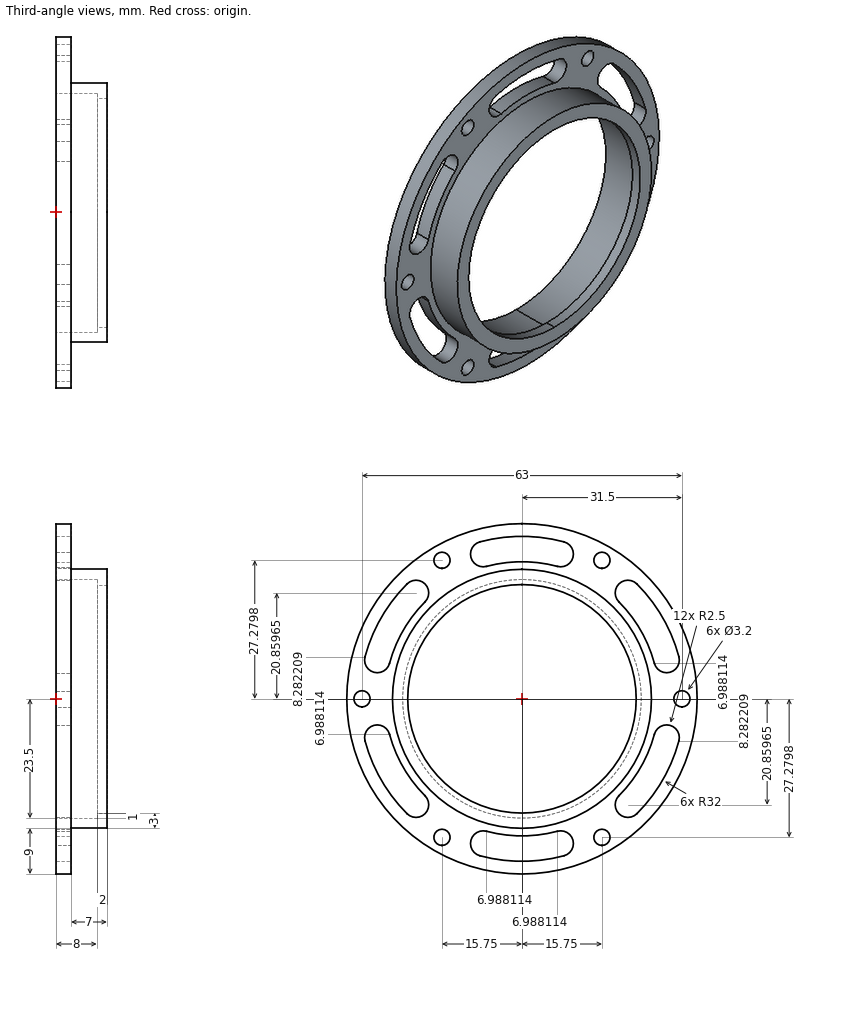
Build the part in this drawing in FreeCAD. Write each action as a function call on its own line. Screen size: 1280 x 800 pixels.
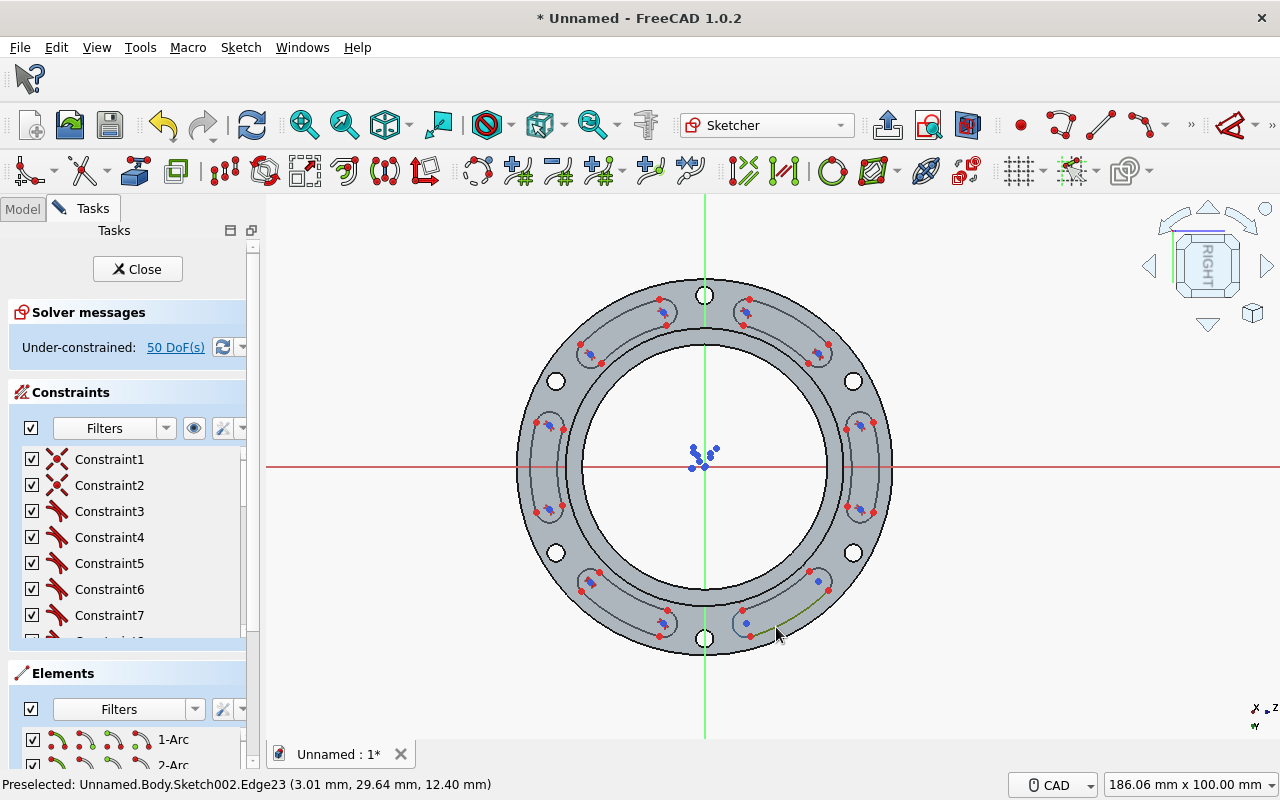
key(t)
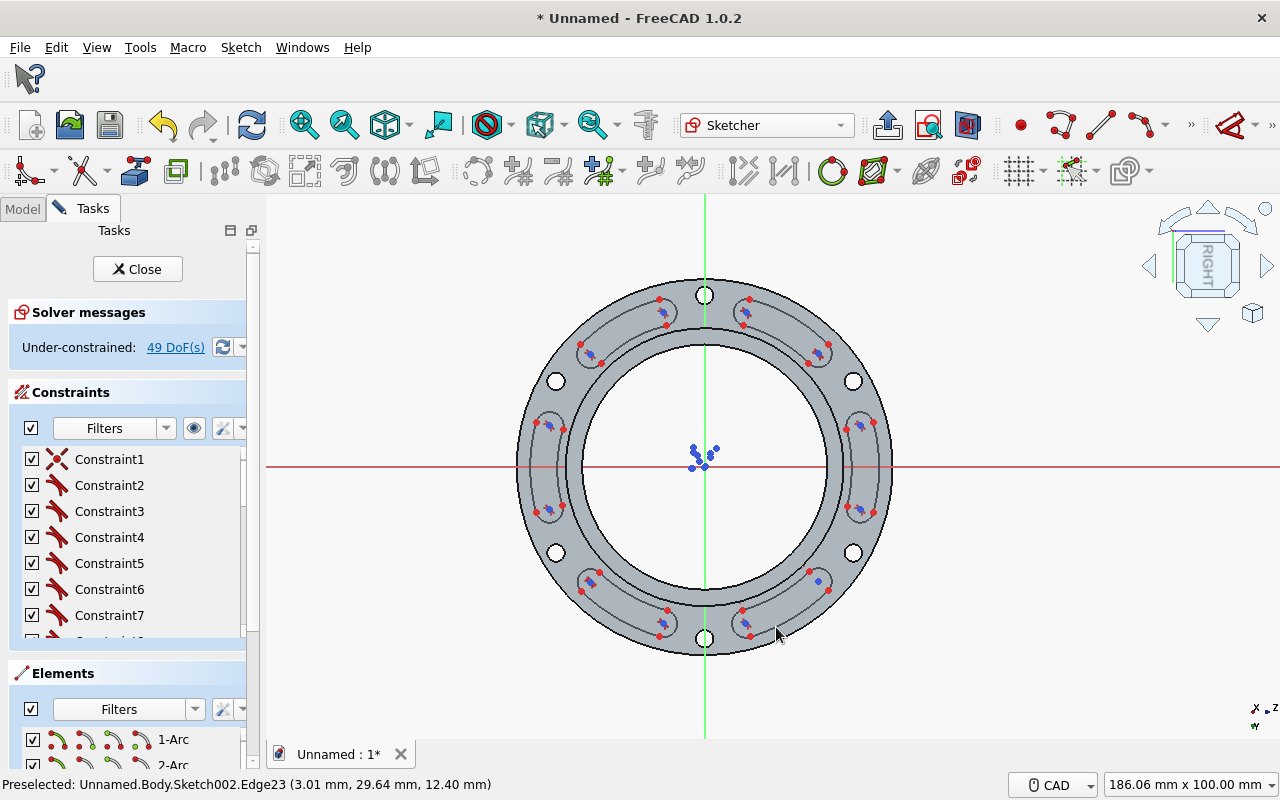
click(776, 627)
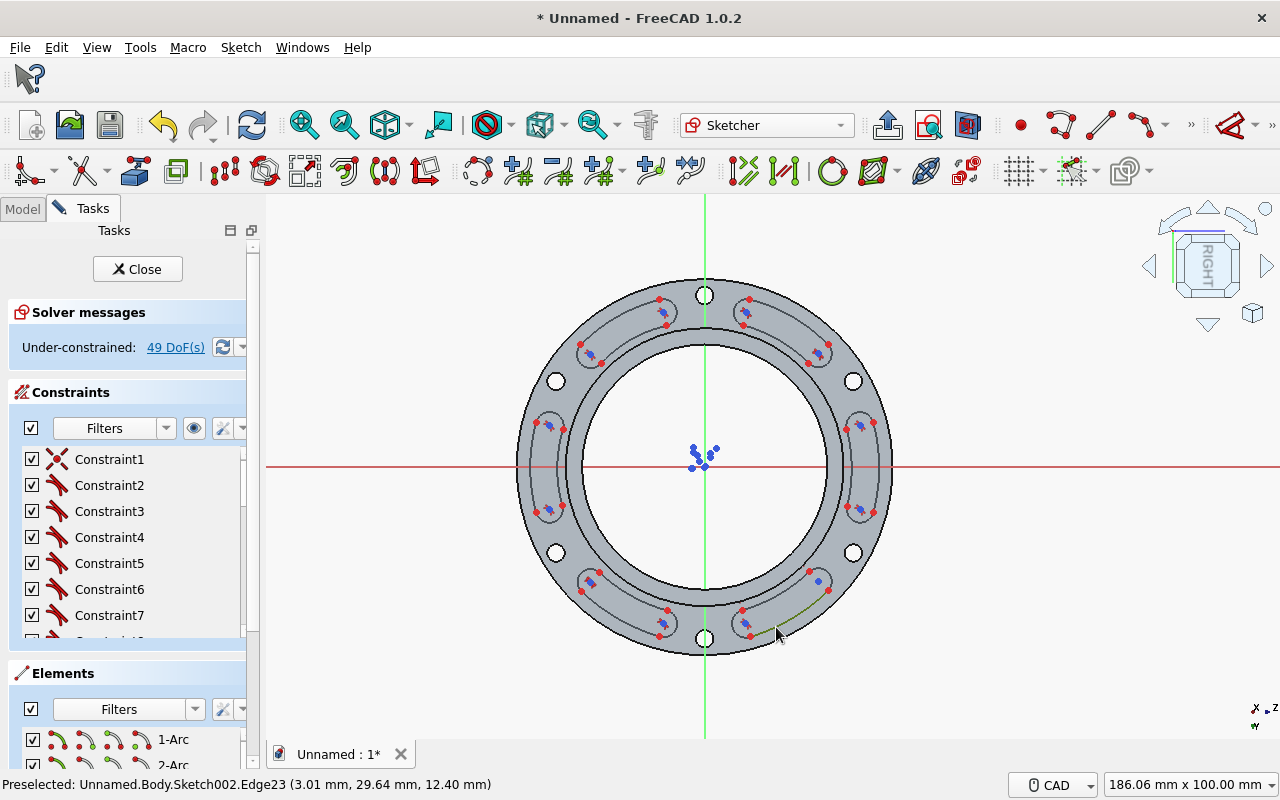
click(832, 579)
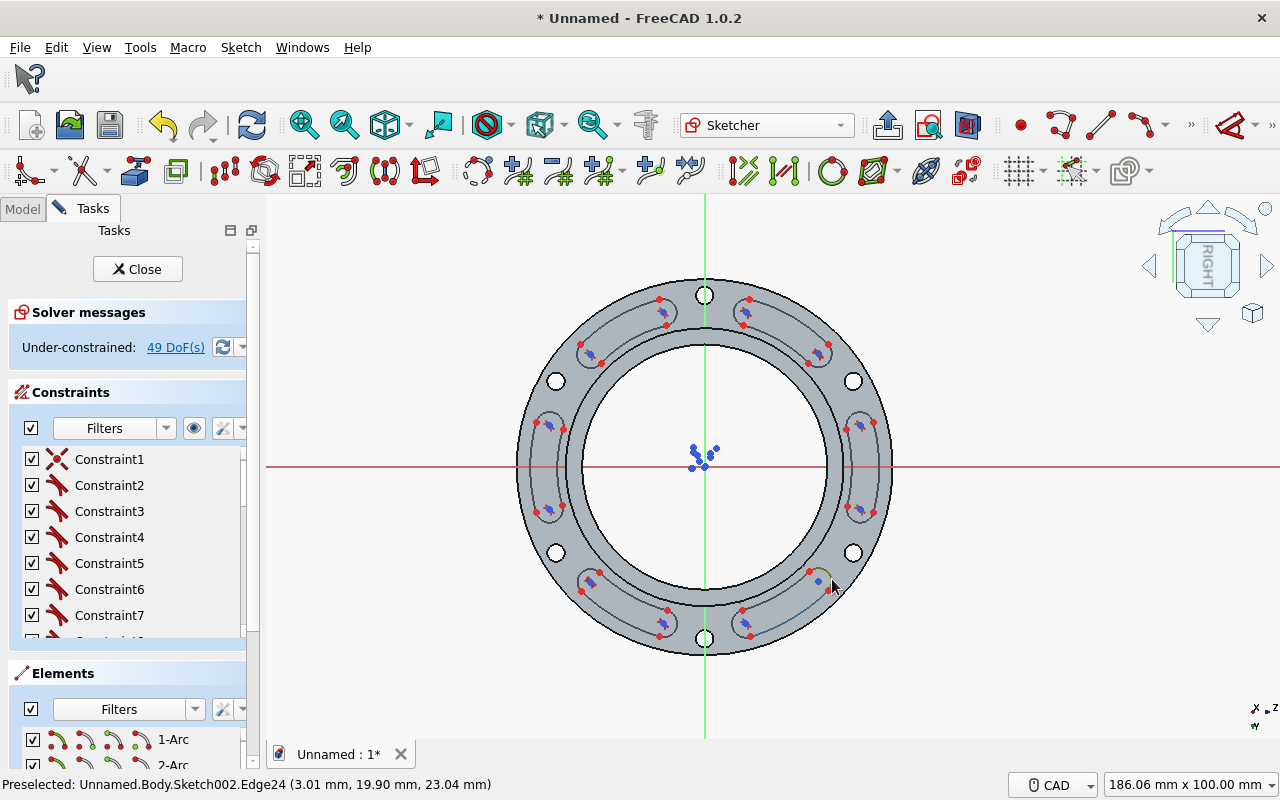
key(t)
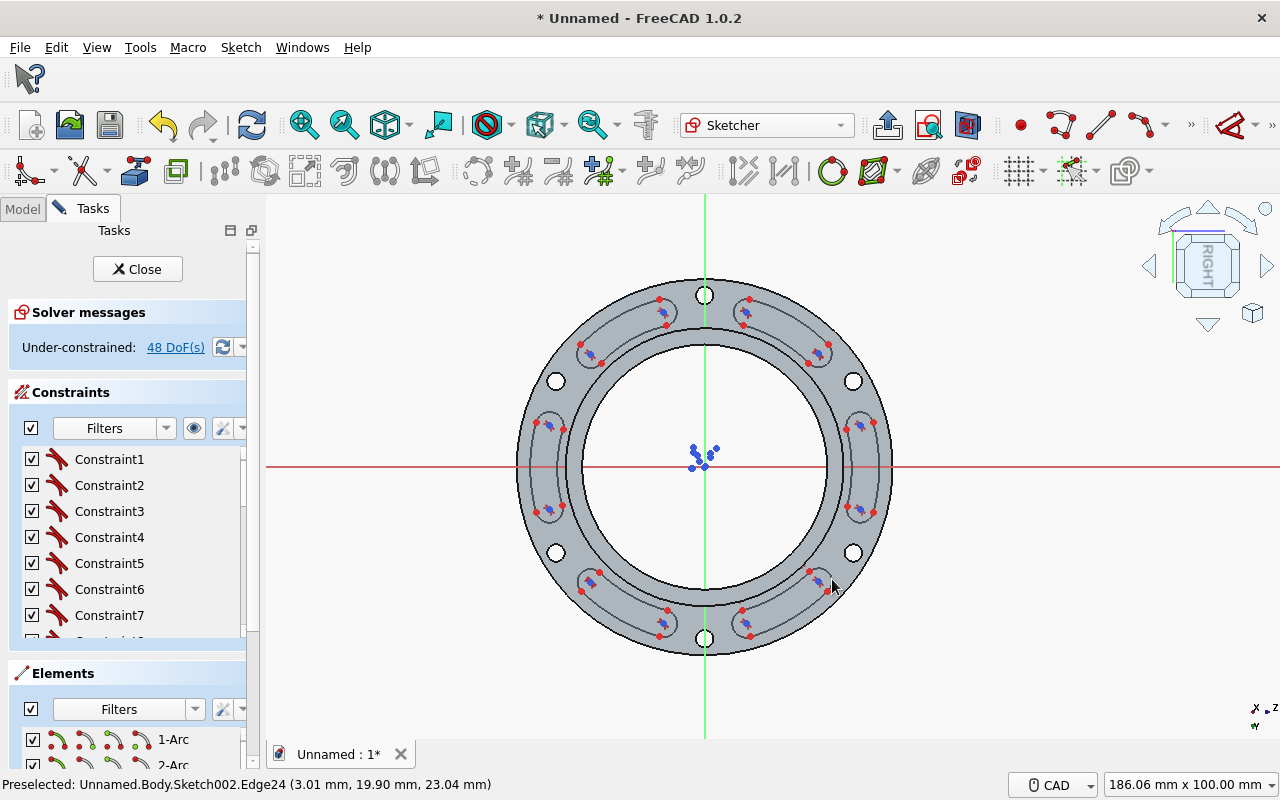
click(603, 609)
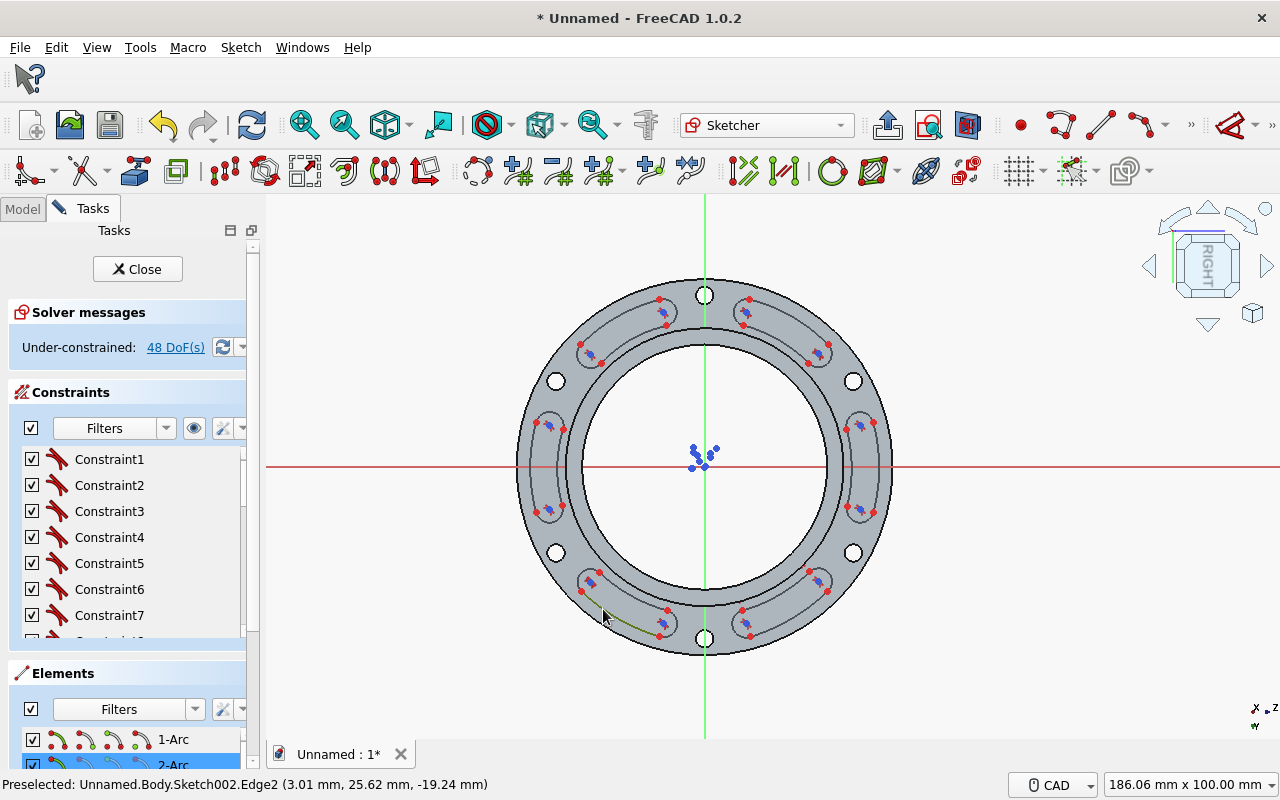
click(618, 587)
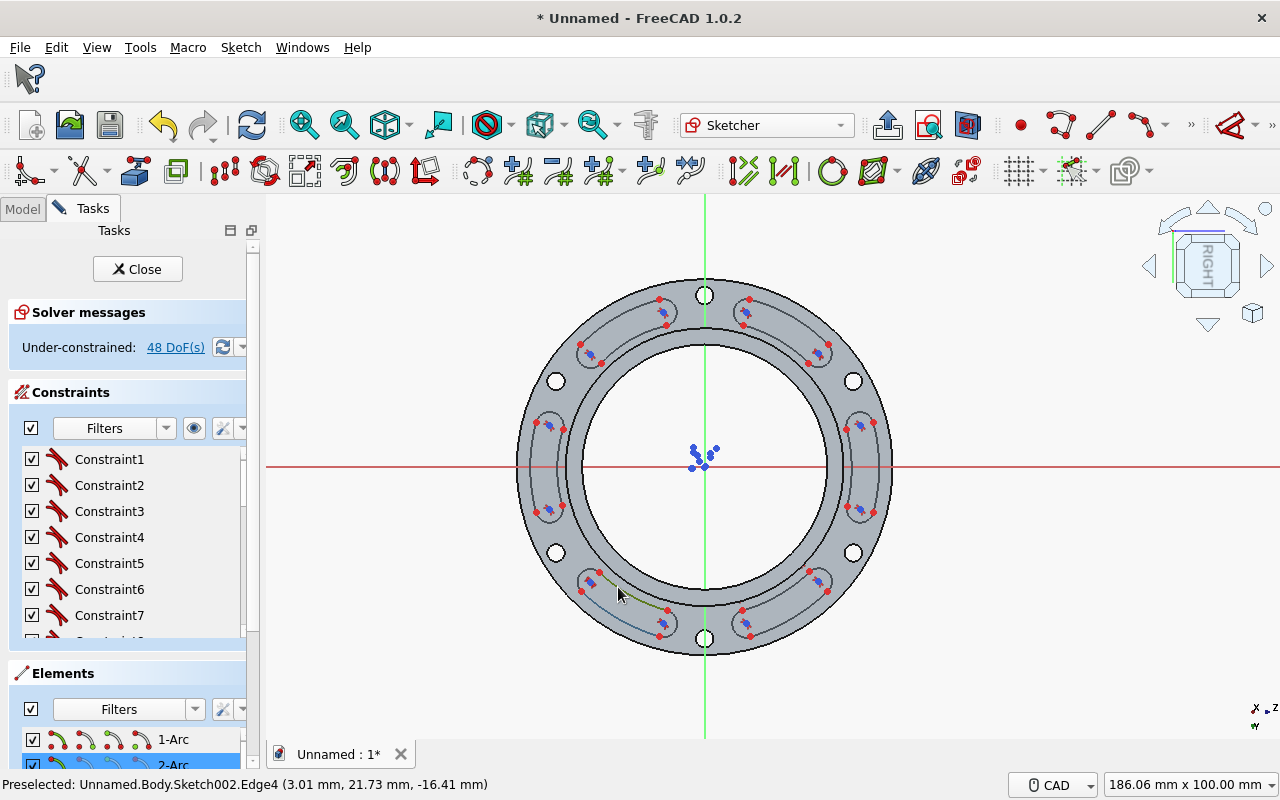
key(c)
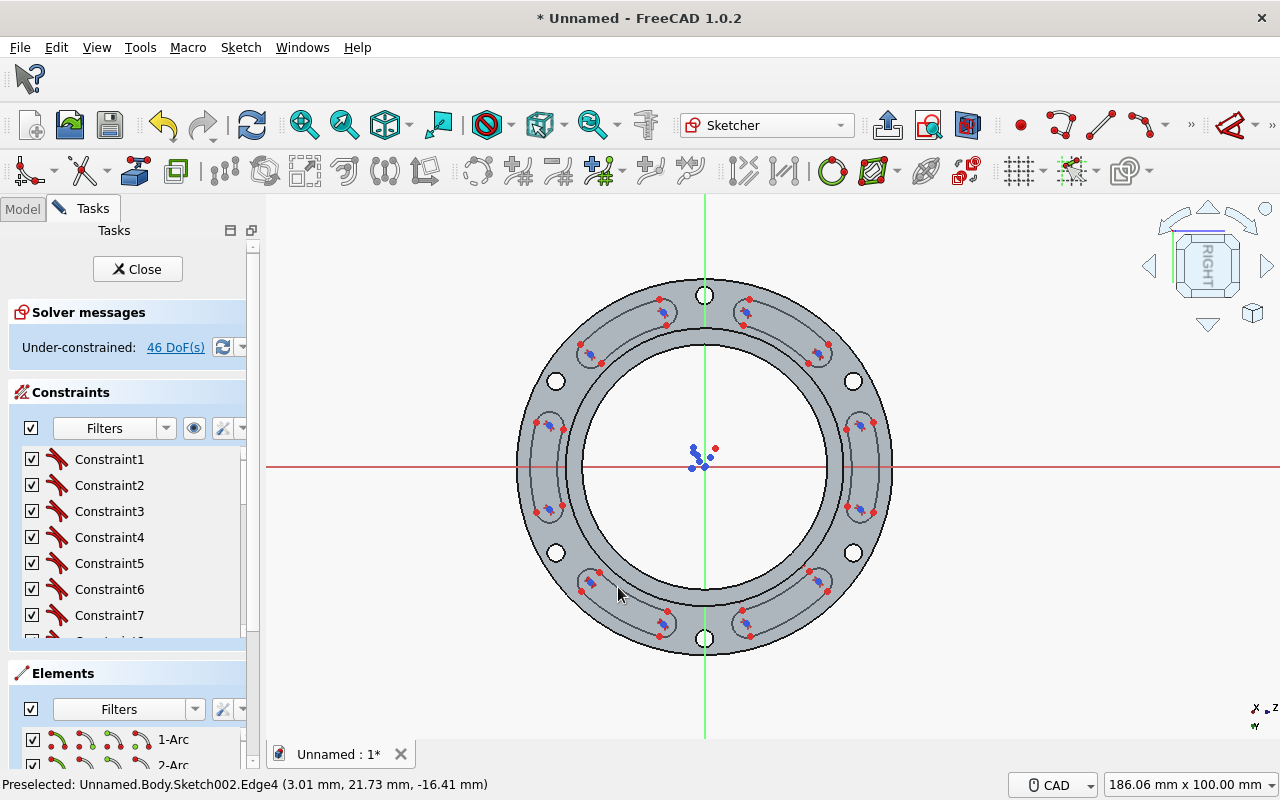
click(603, 609)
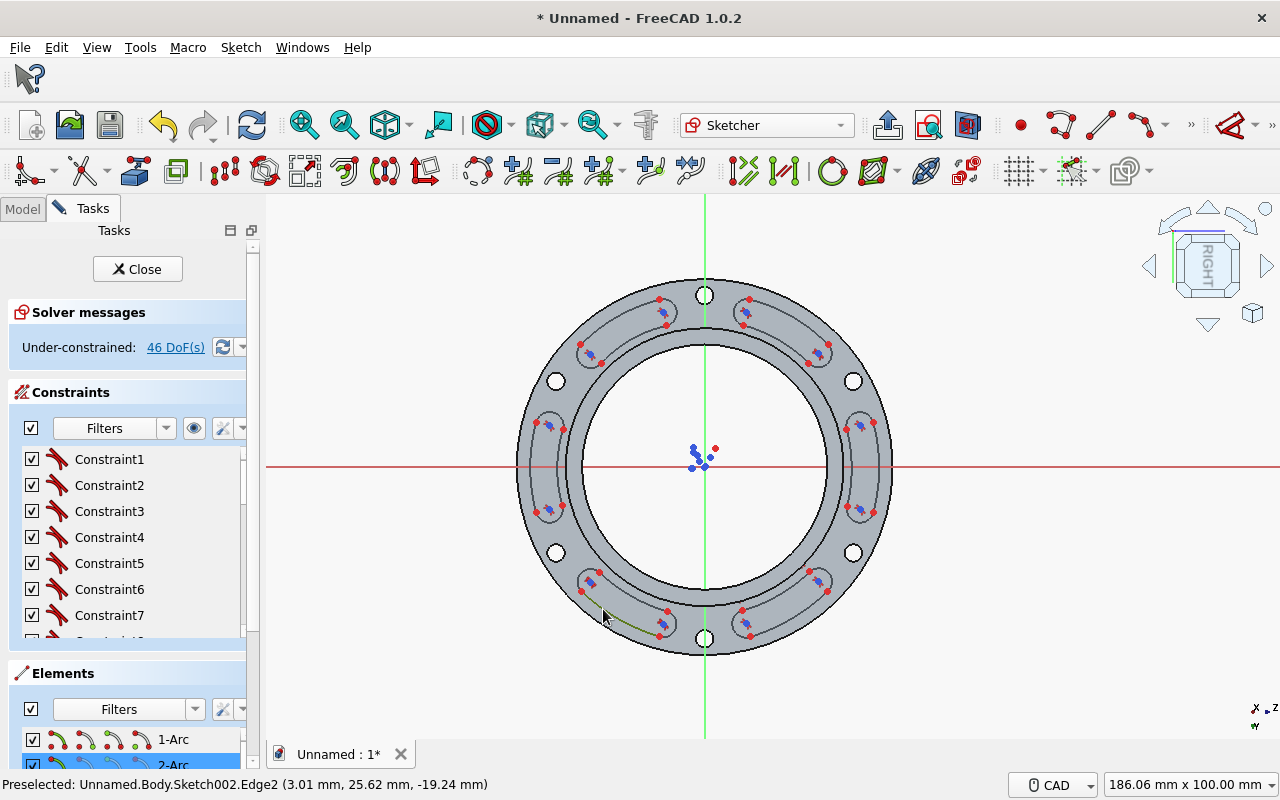
click(558, 452)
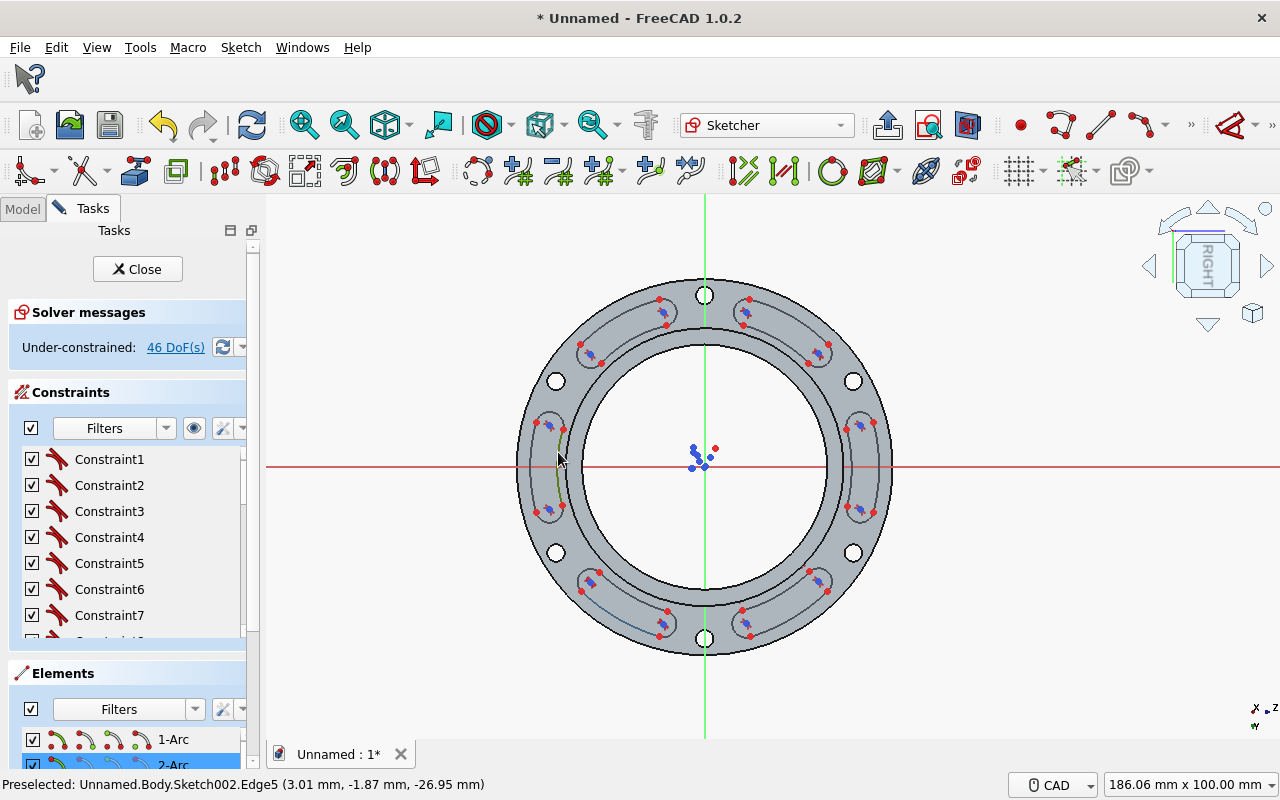
key(c)